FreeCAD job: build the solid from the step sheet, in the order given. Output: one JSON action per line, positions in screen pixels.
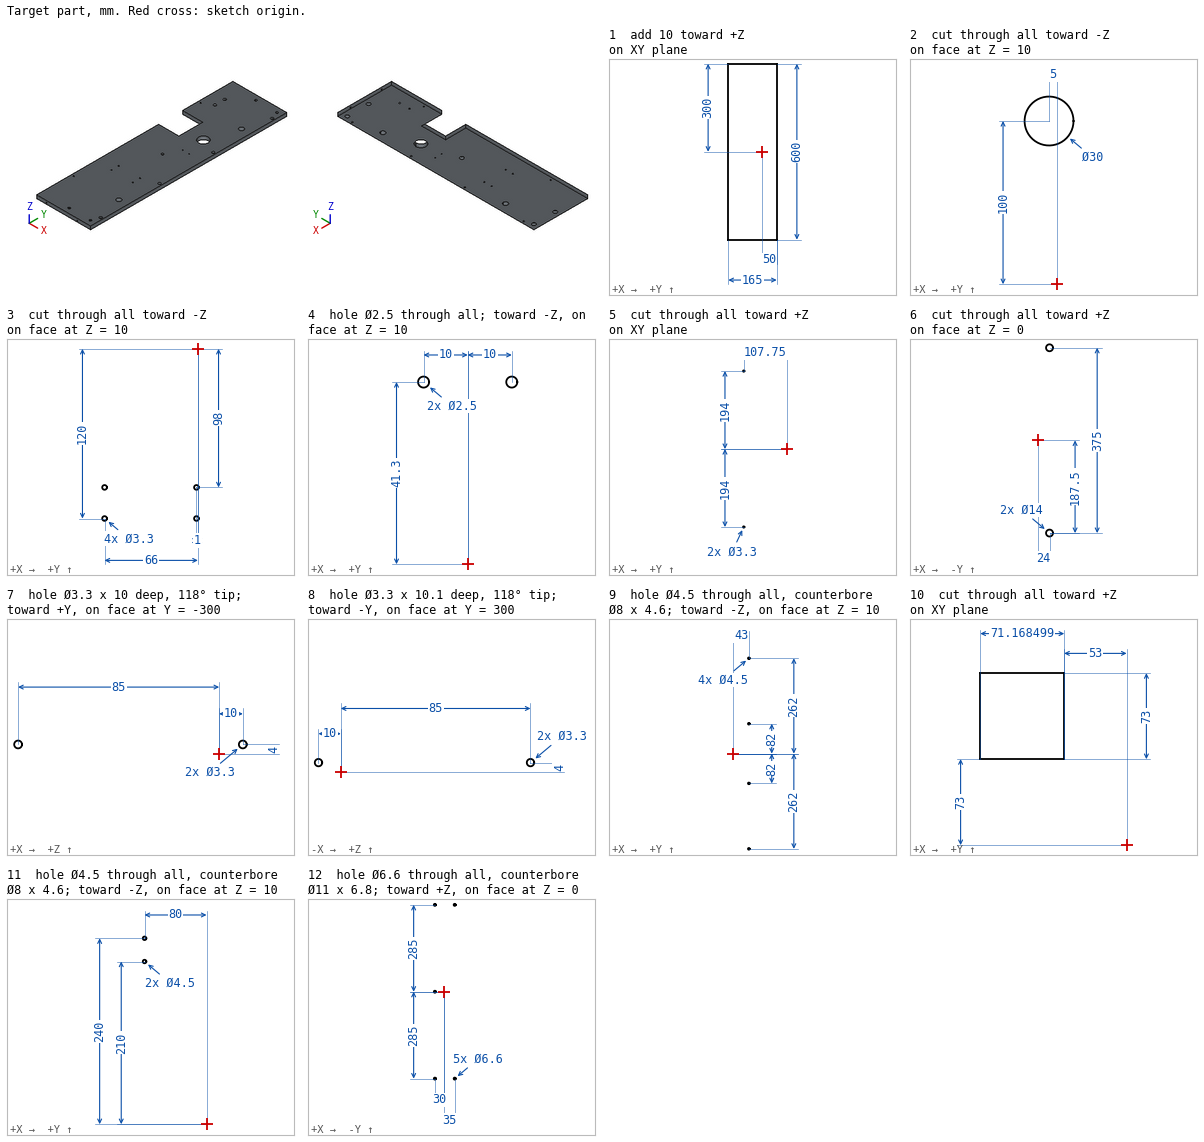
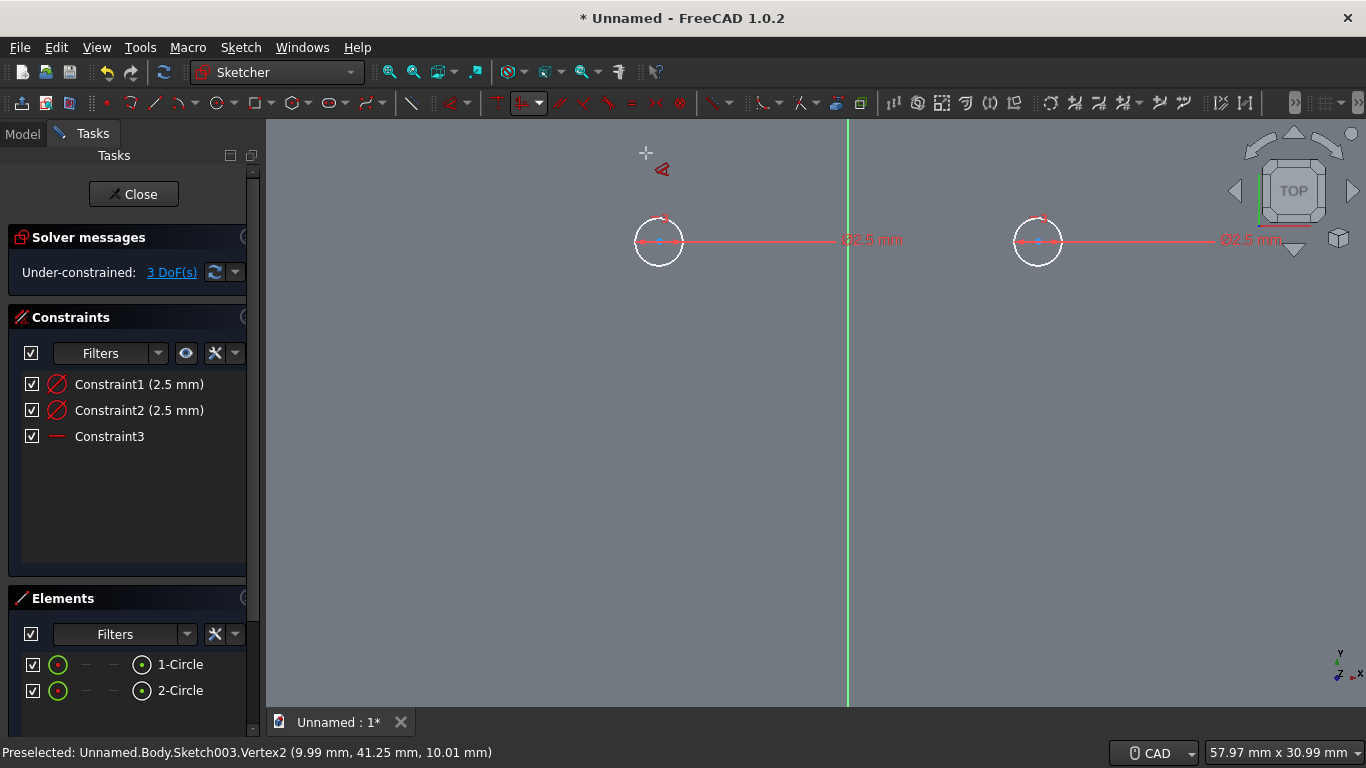
{"action": "left_click", "coordinate": [659, 242]}
{"action": "left_click", "coordinate": [754, 208]}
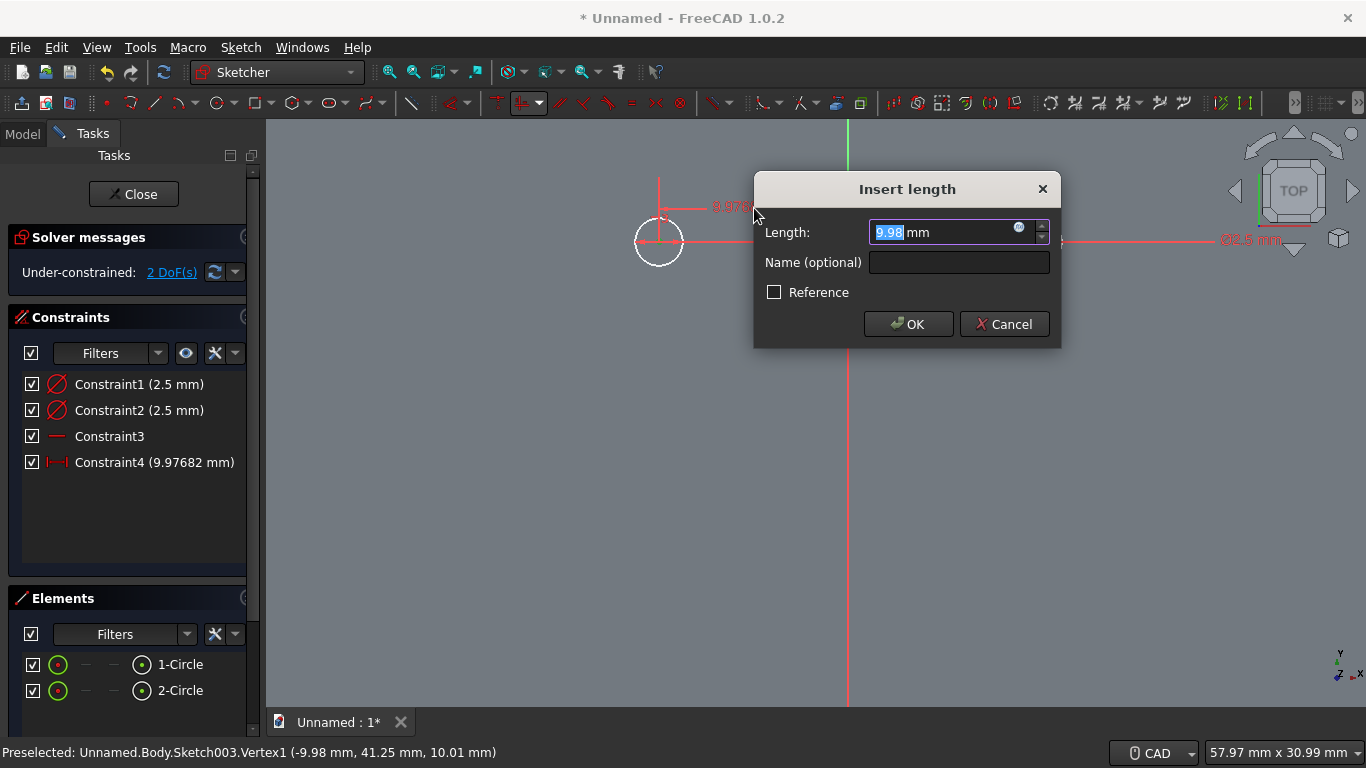
{"action": "type", "text": "10"}
{"action": "key", "text": "Return"}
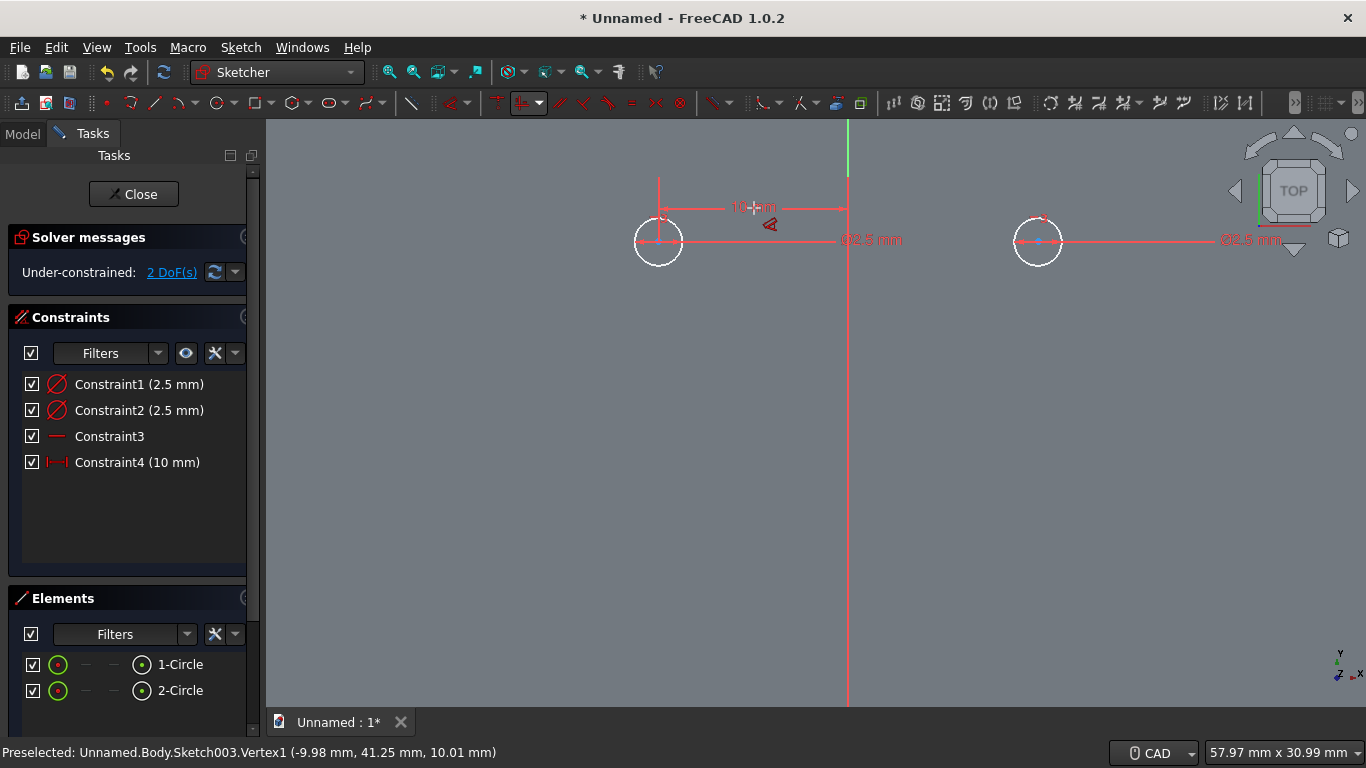
{"action": "left_click", "coordinate": [1038, 242]}
{"action": "left_click", "coordinate": [943, 208]}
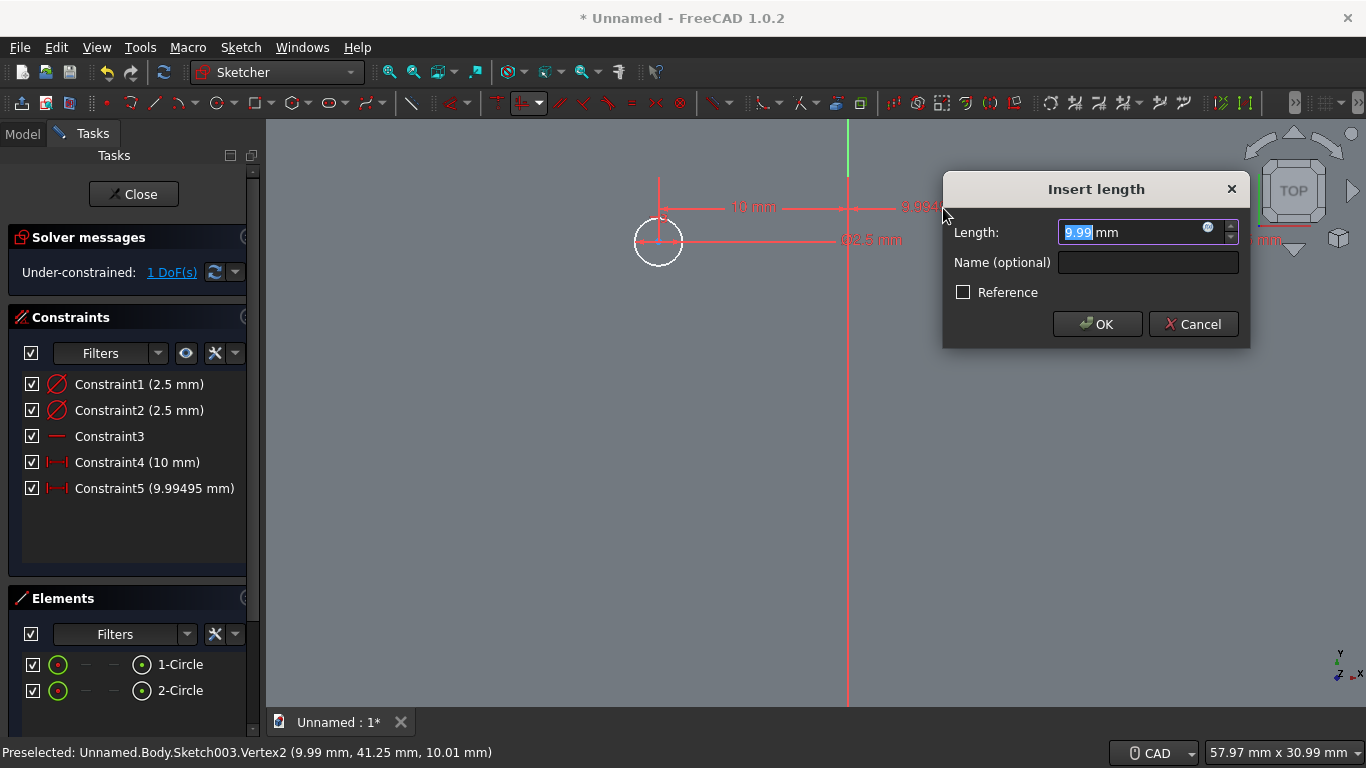
{"action": "type", "text": "10"}
{"action": "key", "text": "Return"}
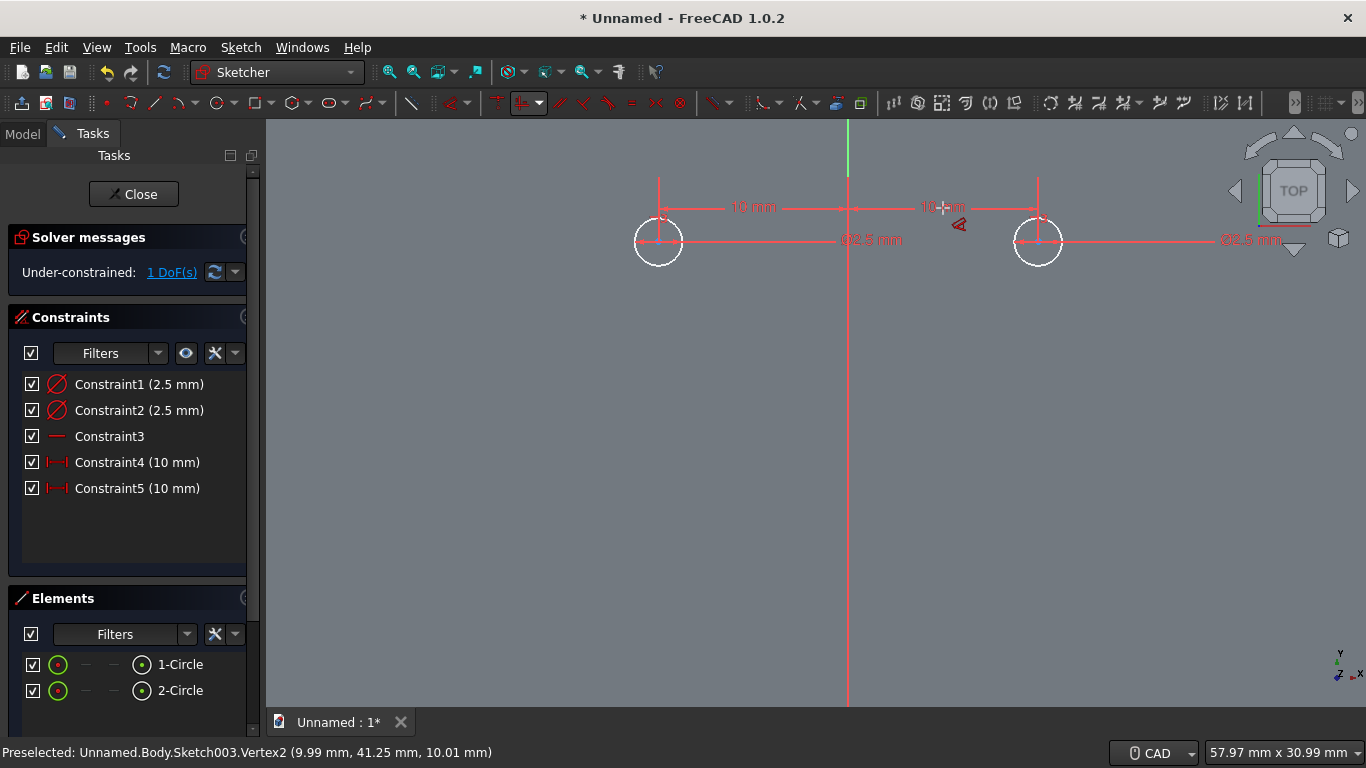
{"action": "left_click", "coordinate": [659, 242]}
{"action": "left_click", "coordinate": [625, 461]}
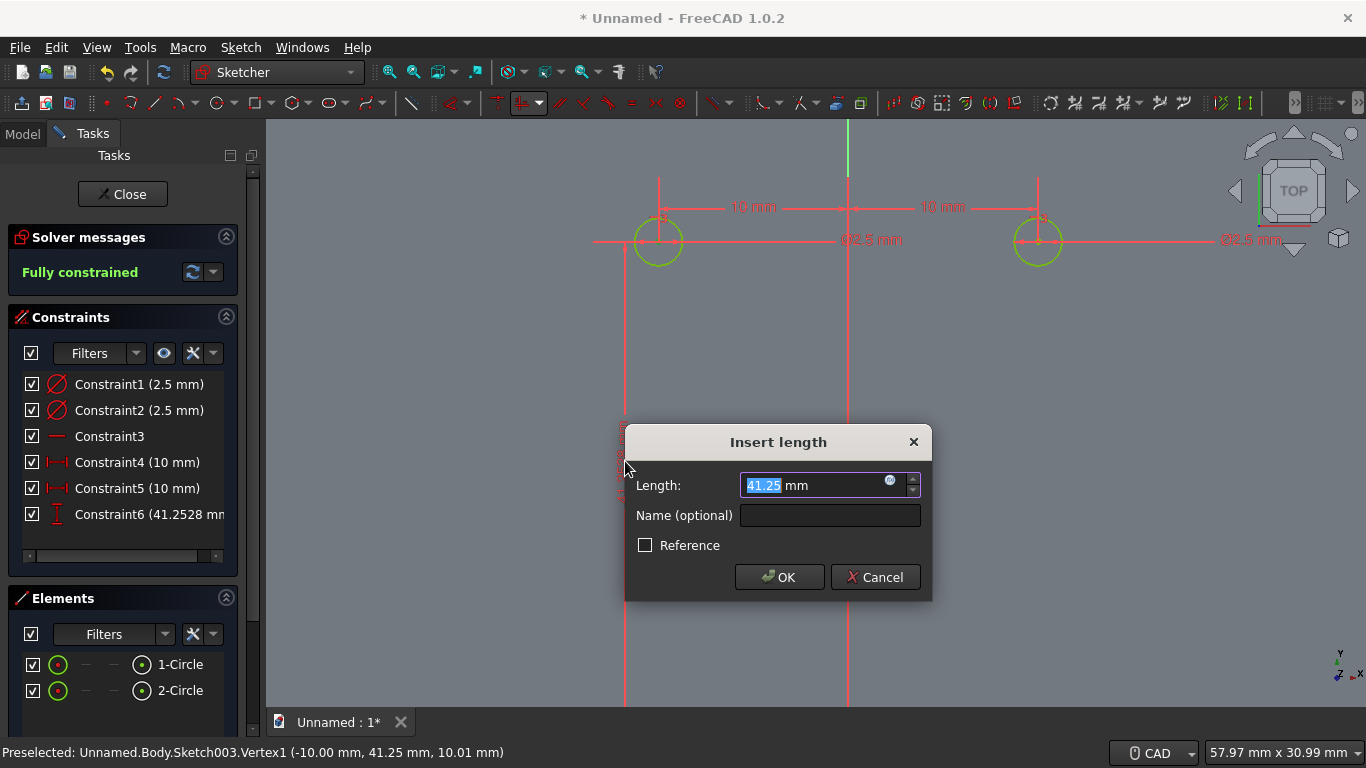
{"action": "type", "text": "41.3"}
{"action": "key", "text": "Return"}
{"action": "key", "text": "Escape"}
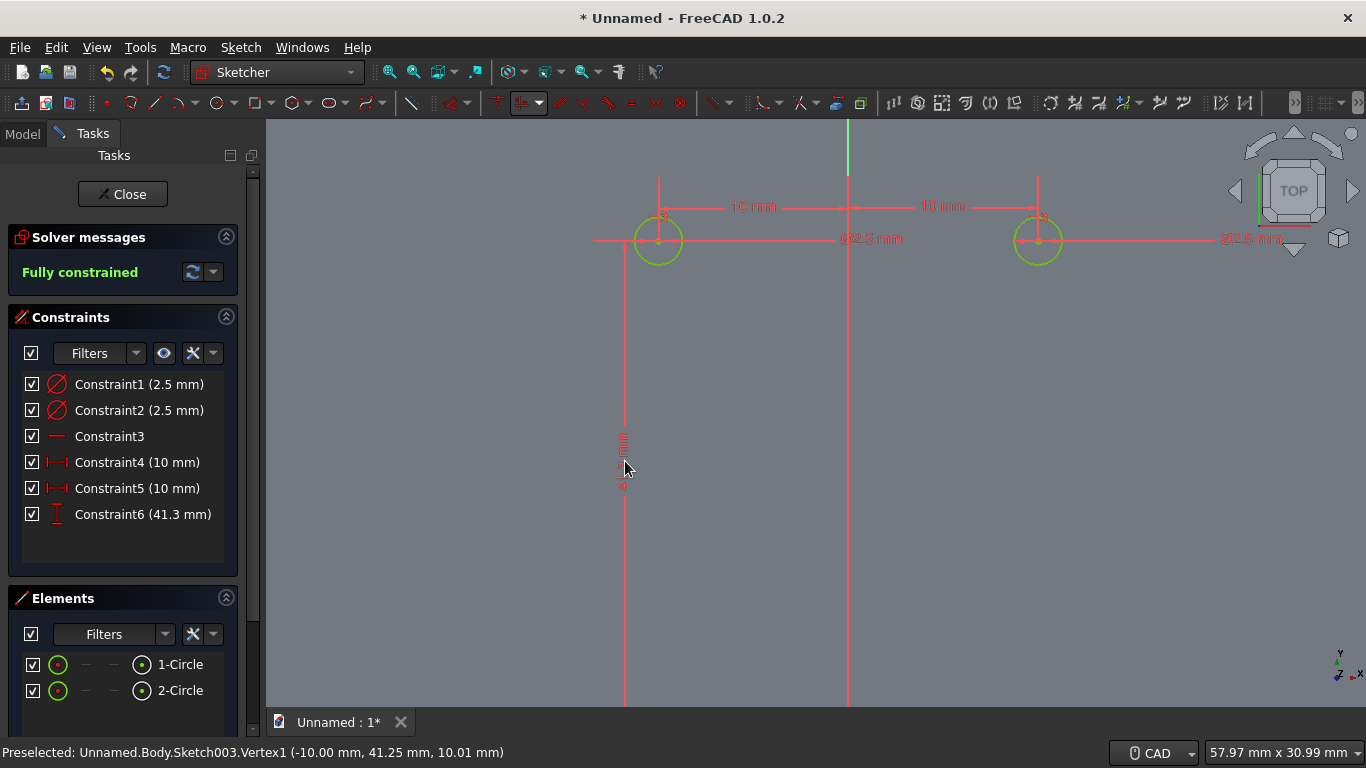
{"action": "left_click", "coordinate": [123, 194]}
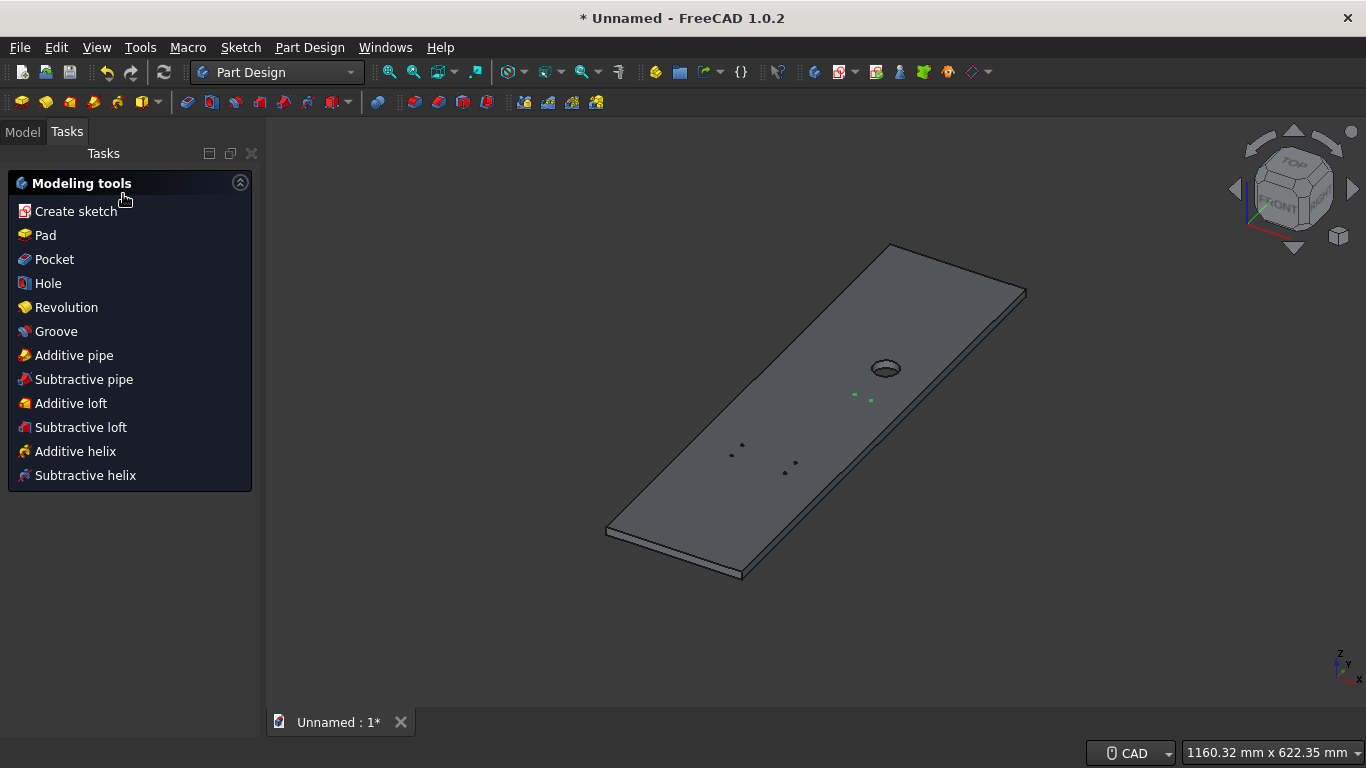
{"action": "left_click", "coordinate": [212, 102]}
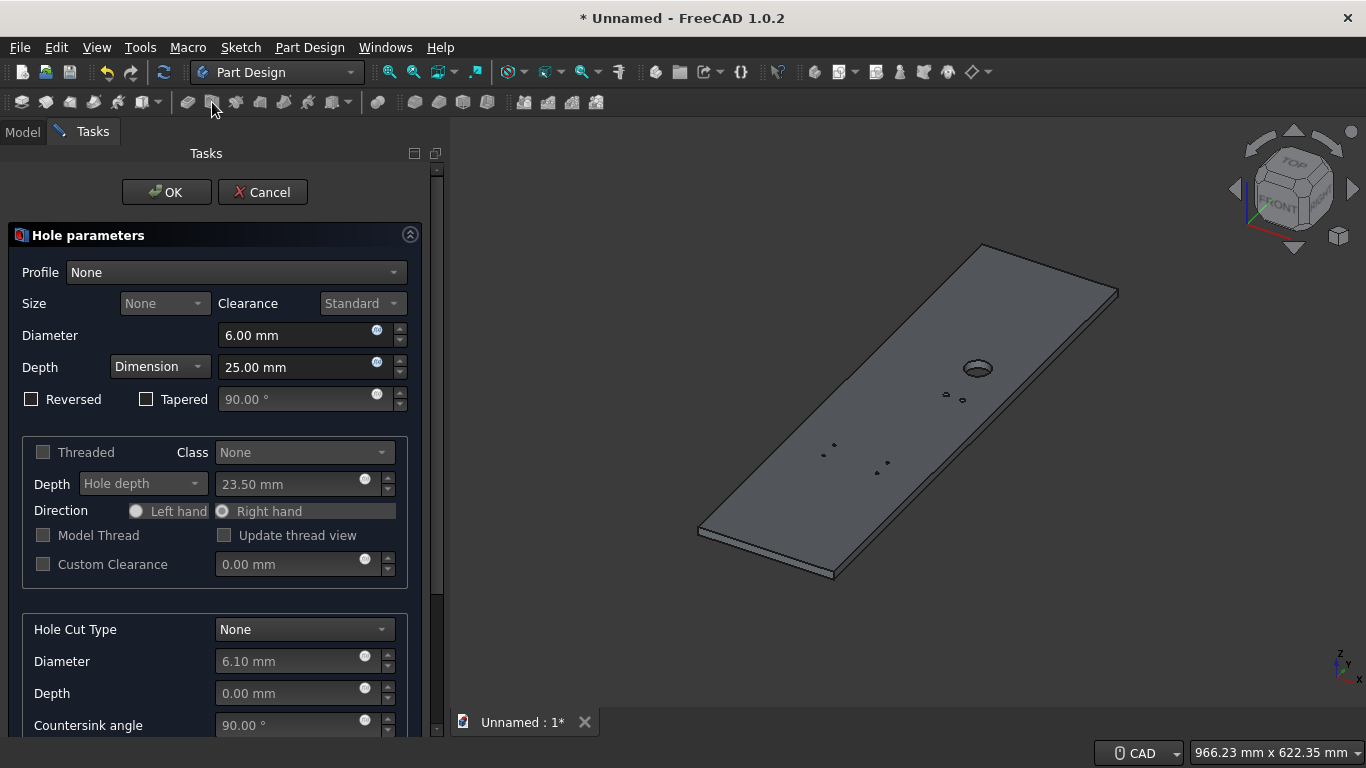
{"action": "triple_click", "coordinate": [305, 335]}